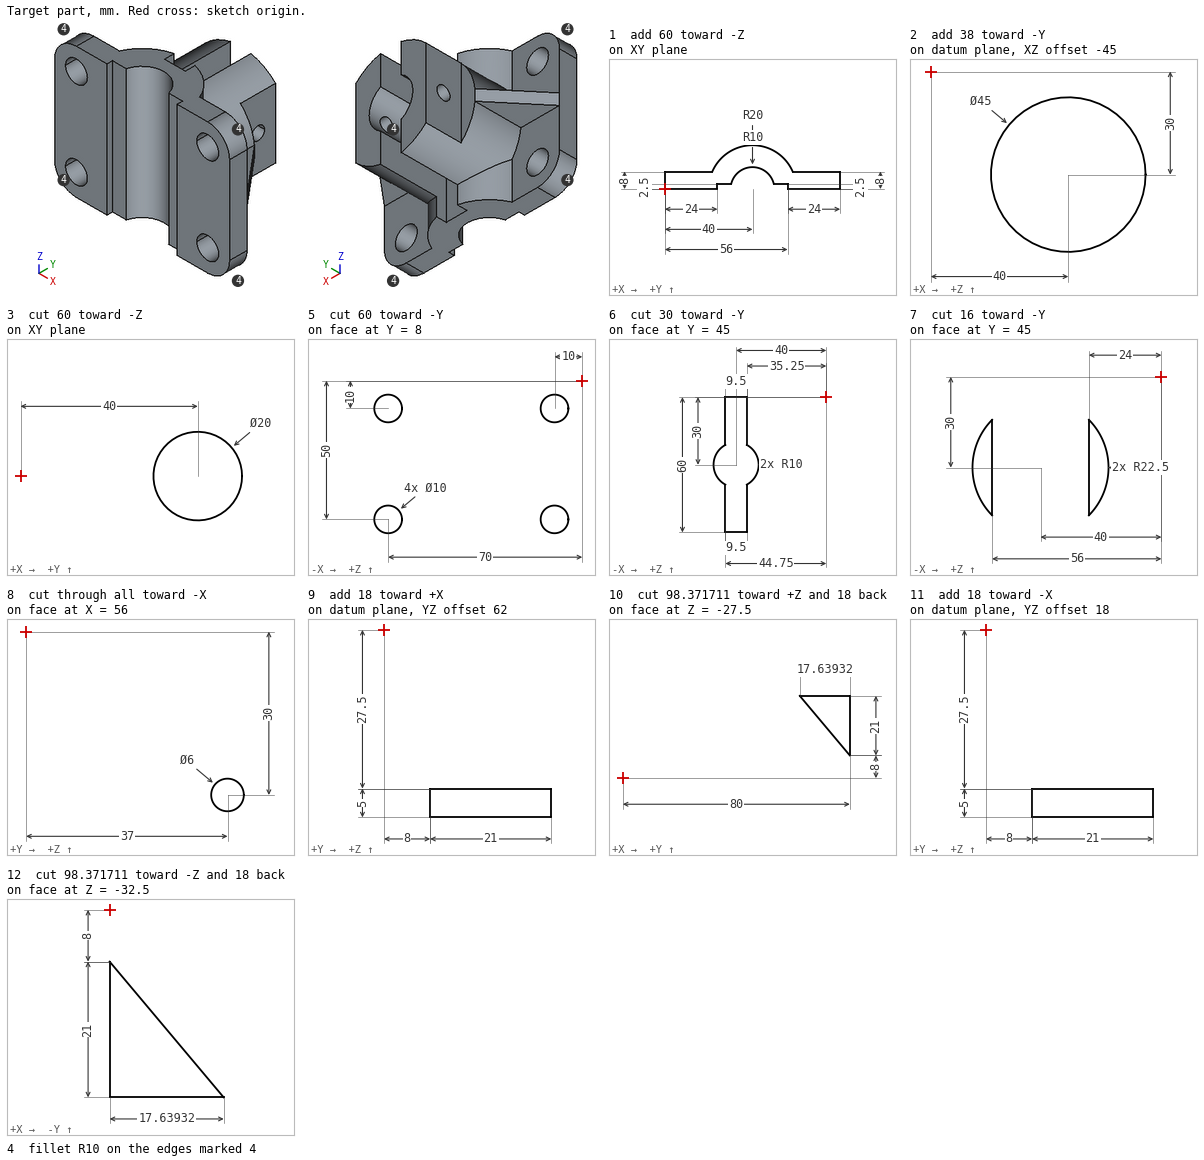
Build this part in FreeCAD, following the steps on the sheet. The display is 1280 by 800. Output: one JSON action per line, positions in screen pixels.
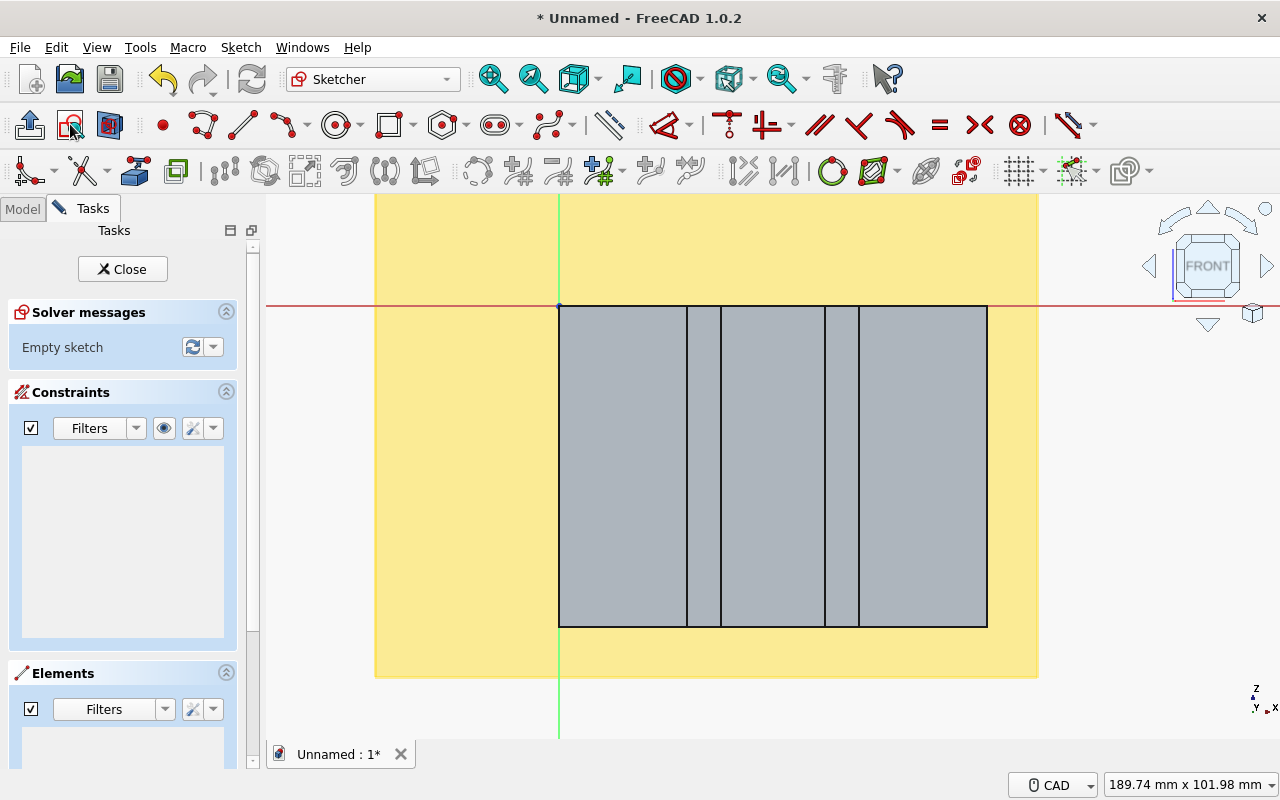
{"action": "left_click", "coordinate": [110, 126]}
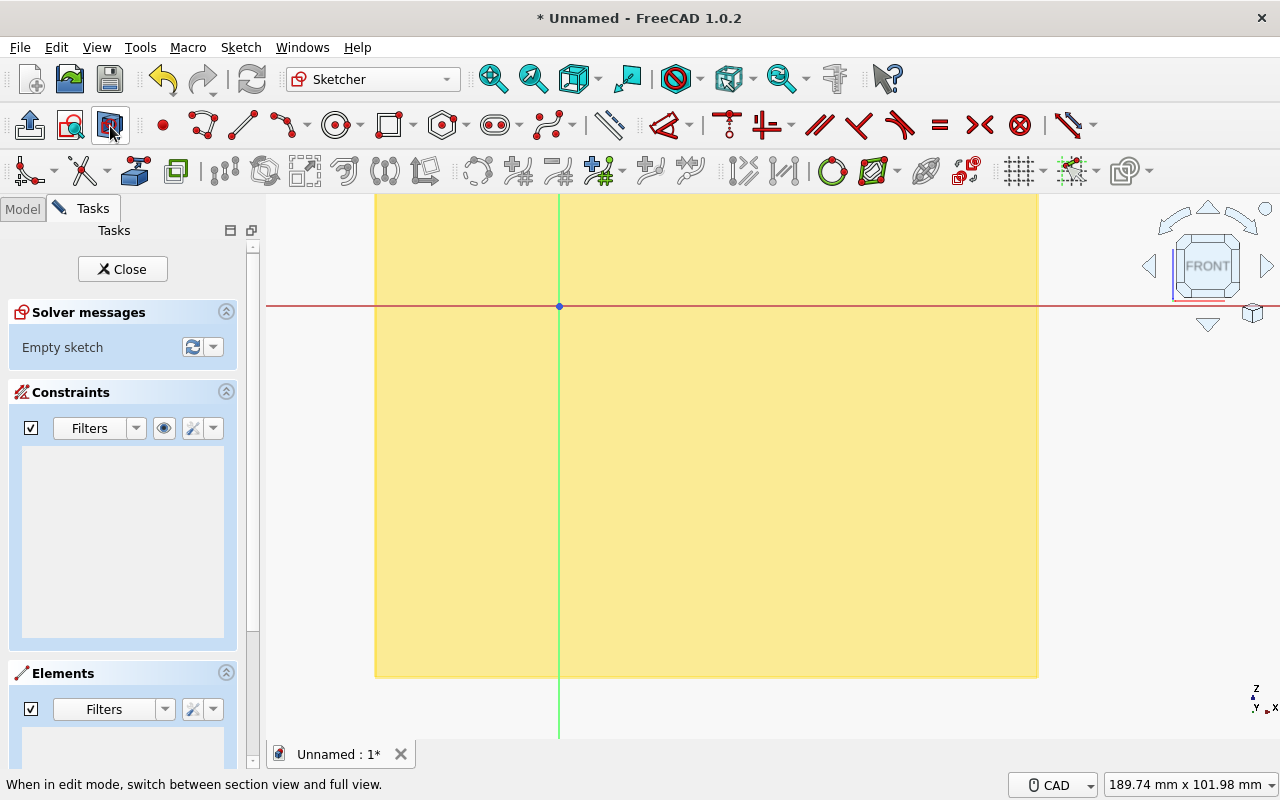
{"action": "left_click", "coordinate": [336, 126]}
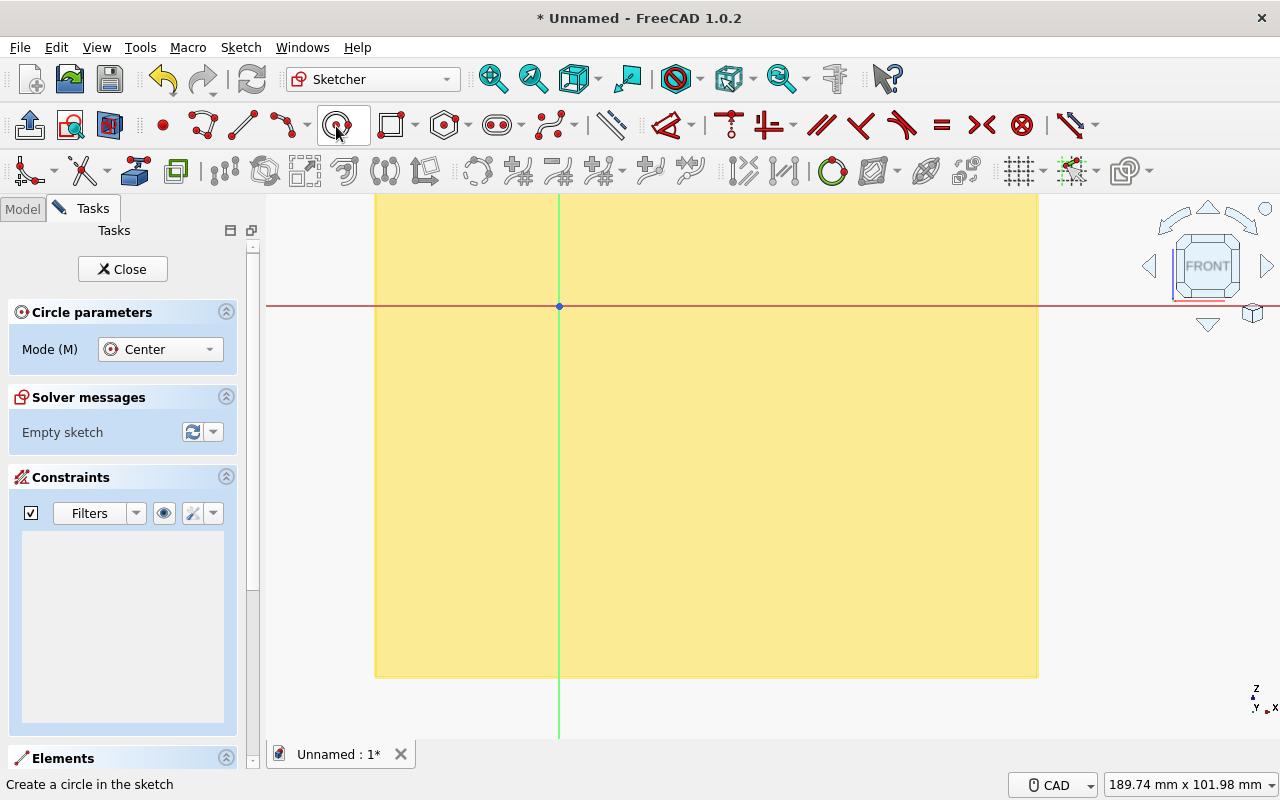
{"action": "left_click", "coordinate": [773, 467]}
{"action": "left_click", "coordinate": [858, 381]}
{"action": "key", "text": "Escape"}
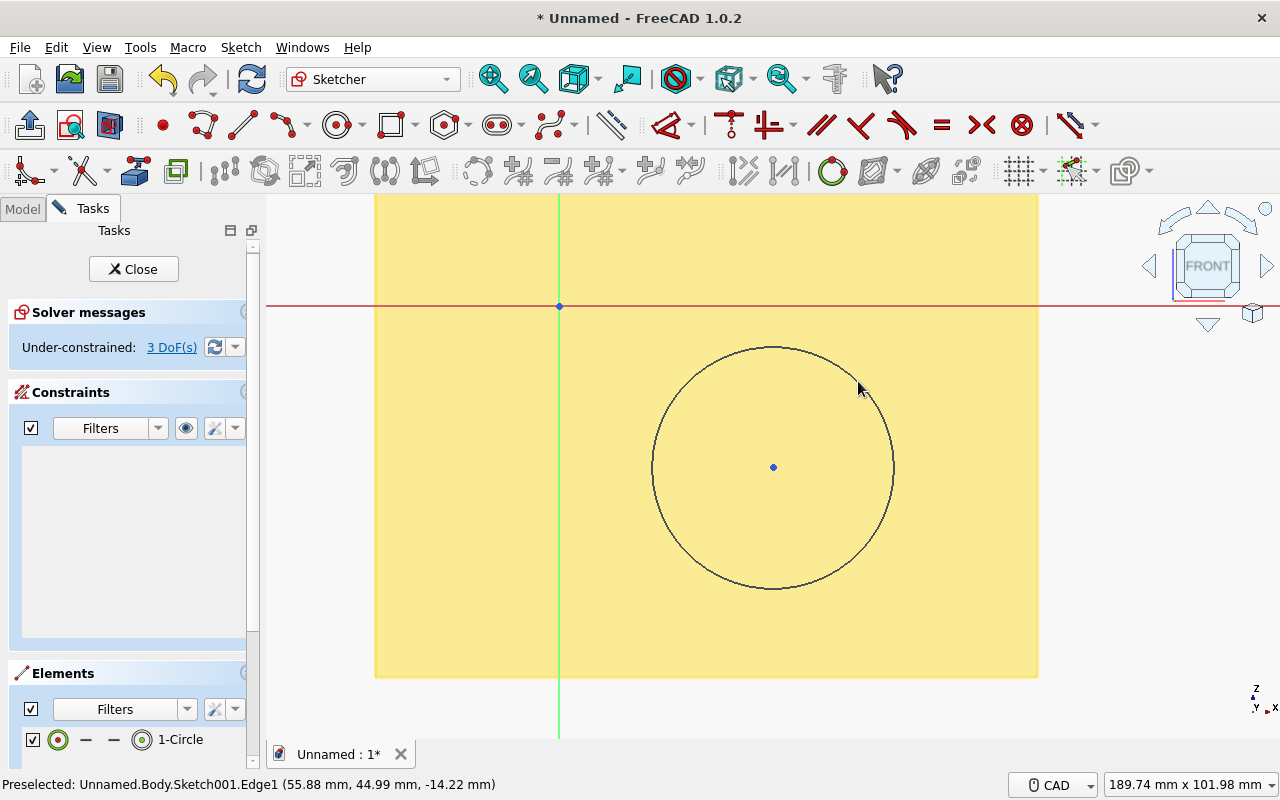
{"action": "left_click", "coordinate": [666, 126]}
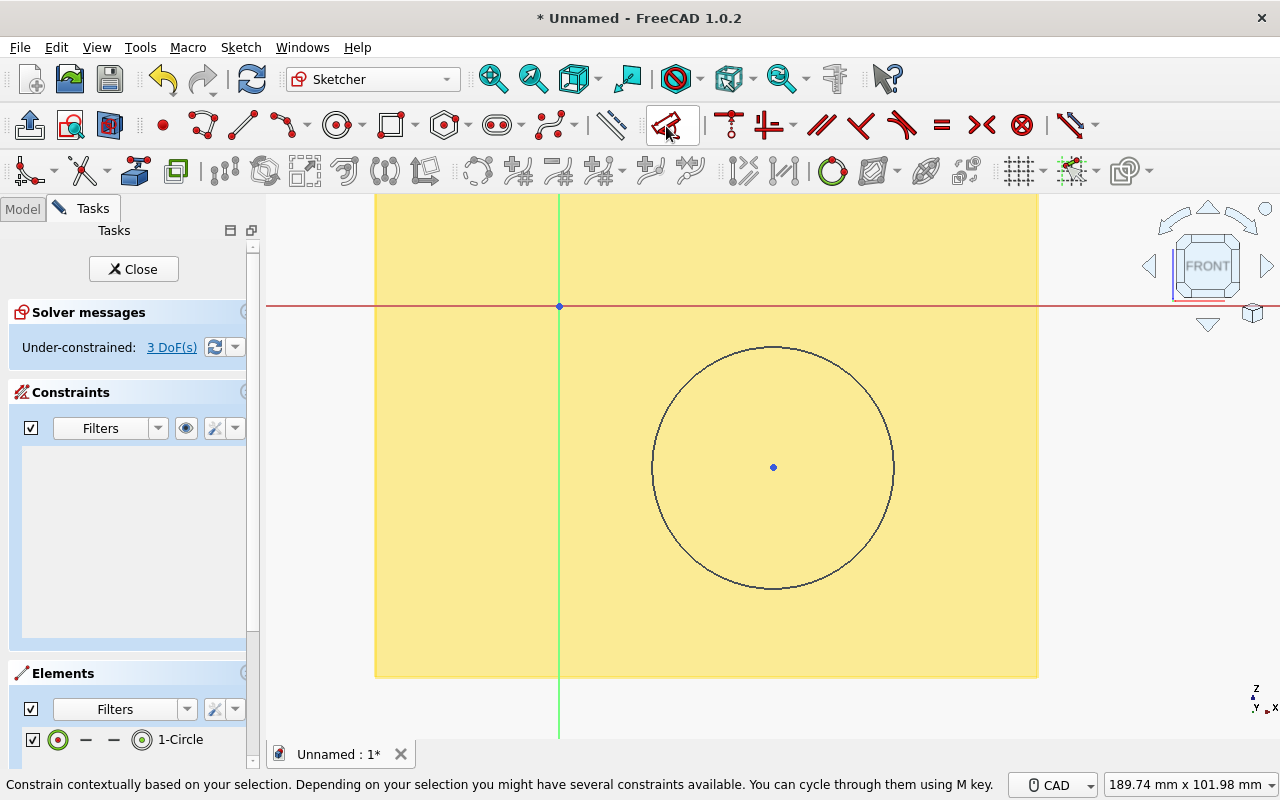
{"action": "left_click", "coordinate": [858, 382]}
{"action": "left_click", "coordinate": [880, 359]}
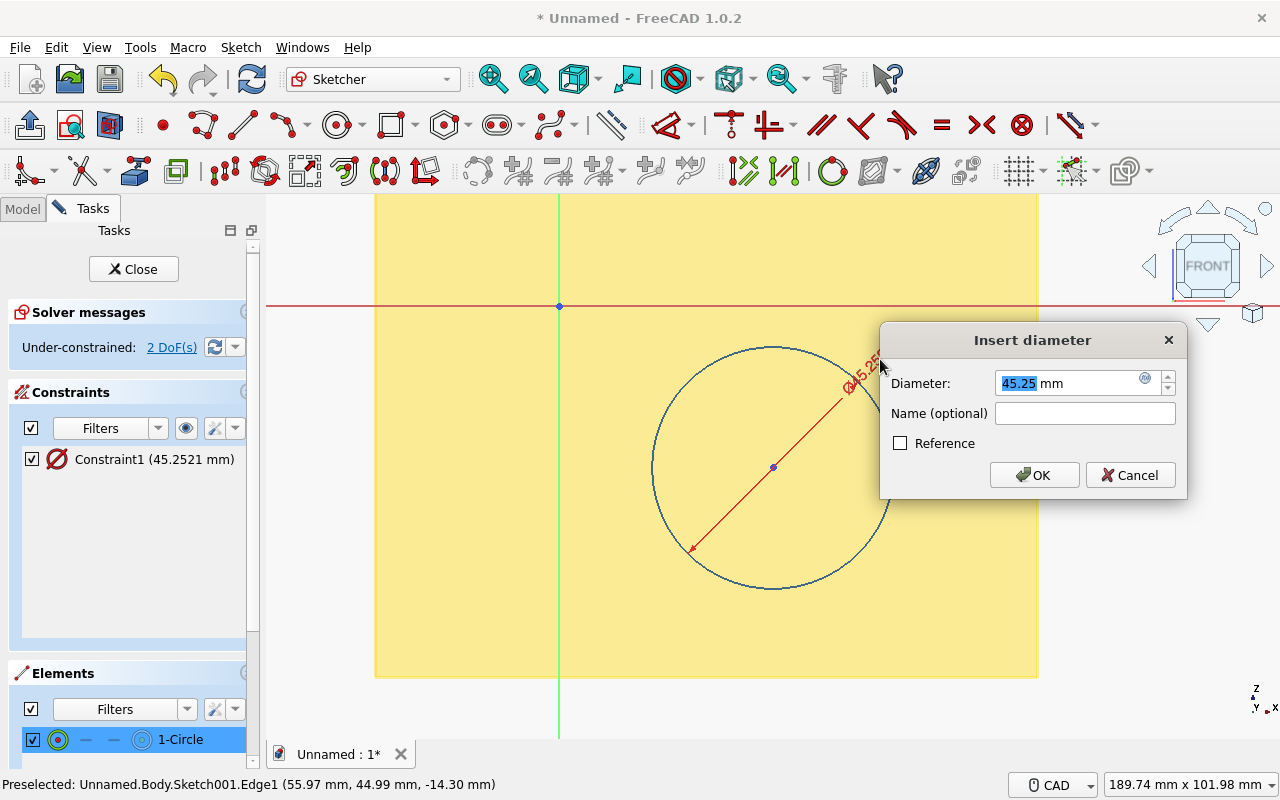
{"action": "type", "text": "45"}
{"action": "key", "text": "Return"}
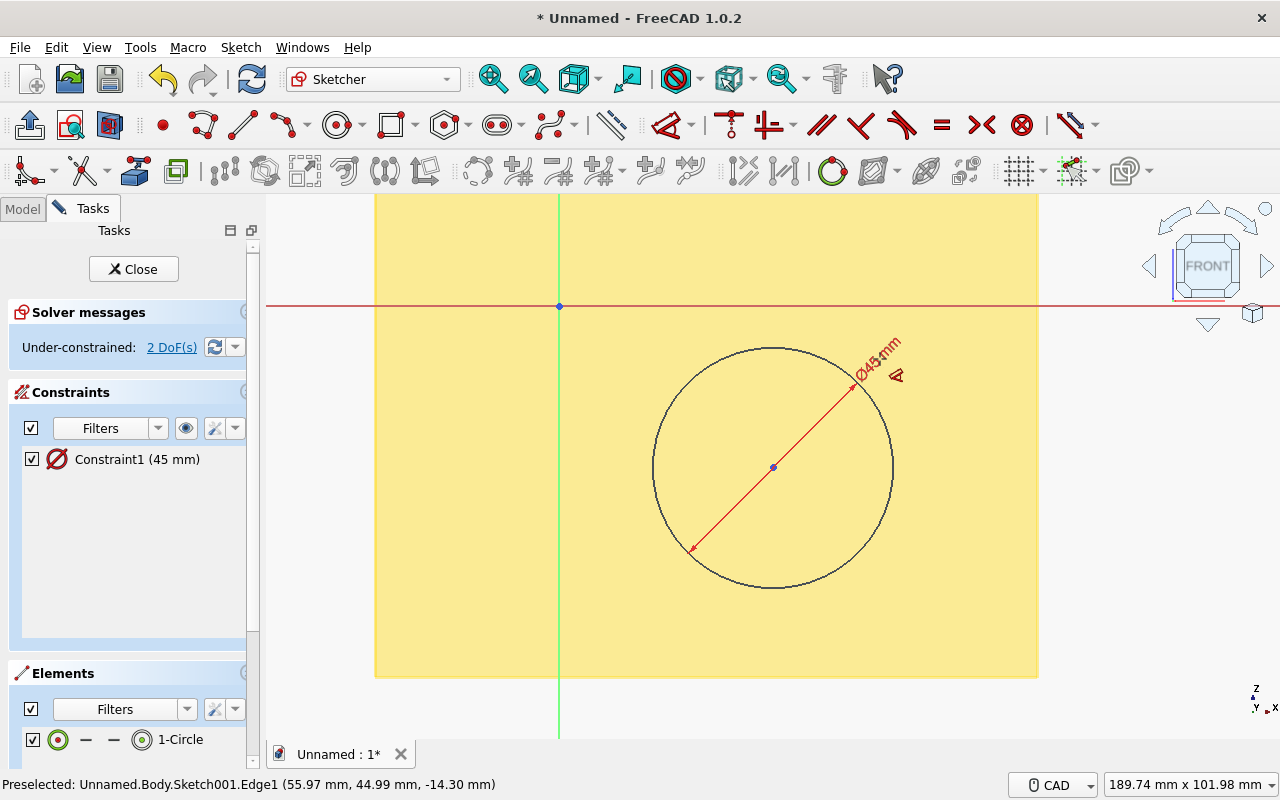
{"action": "left_click", "coordinate": [773, 468]}
{"action": "left_click", "coordinate": [666, 272]}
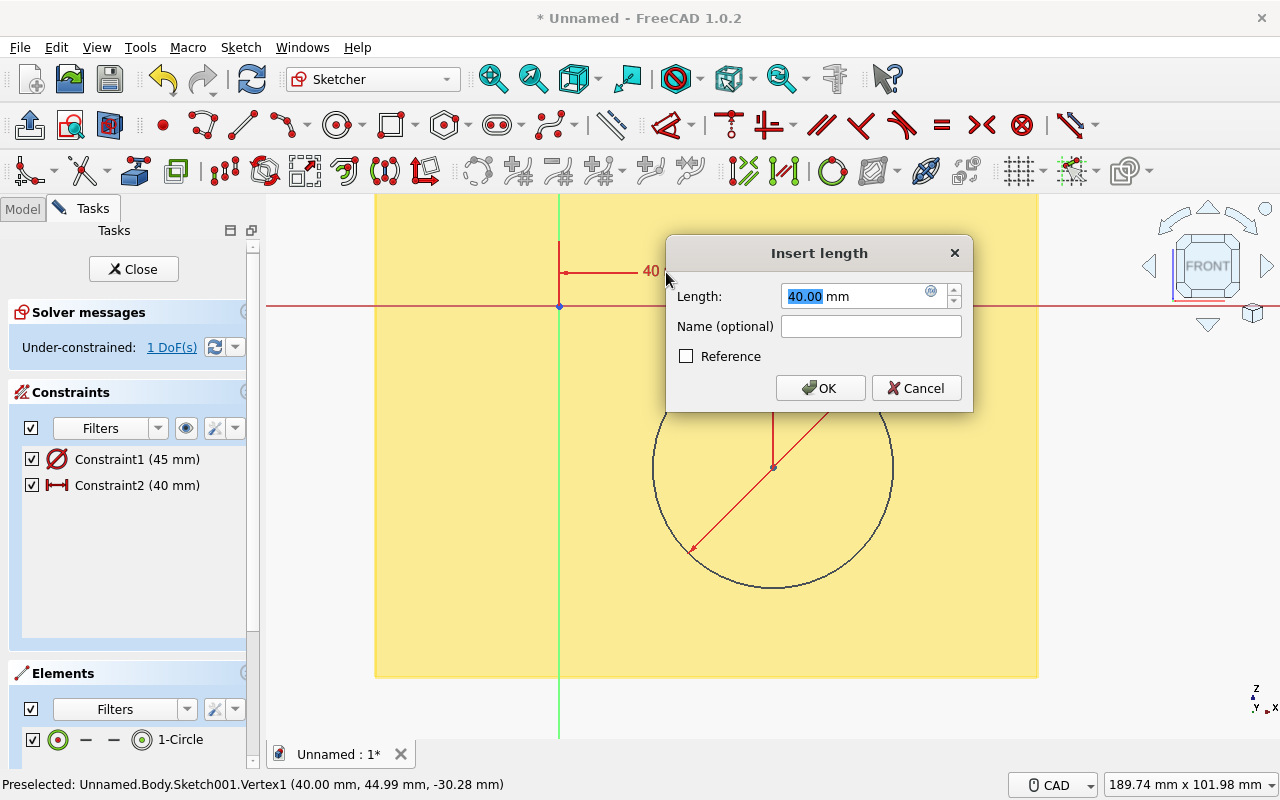
{"action": "type", "text": "40"}
{"action": "key", "text": "Return"}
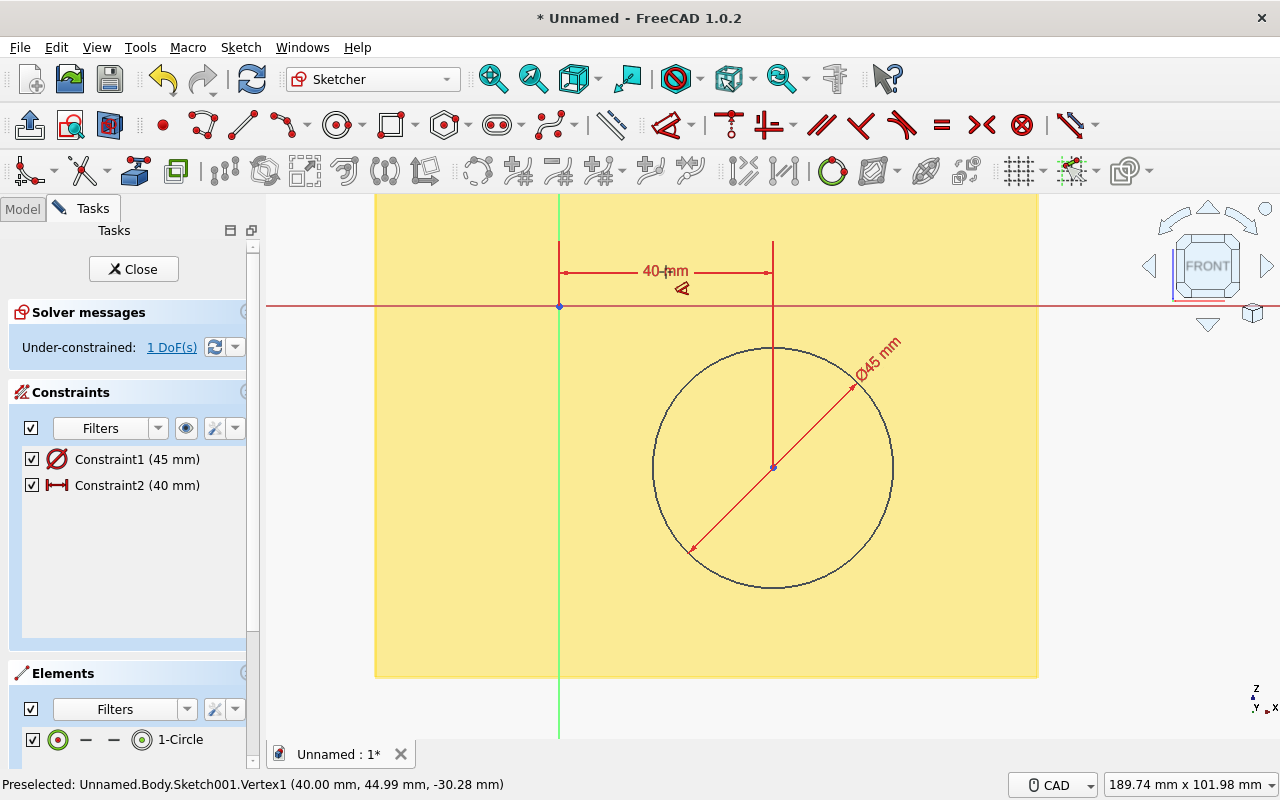
{"action": "left_click", "coordinate": [773, 468]}
{"action": "left_click", "coordinate": [525, 387]}